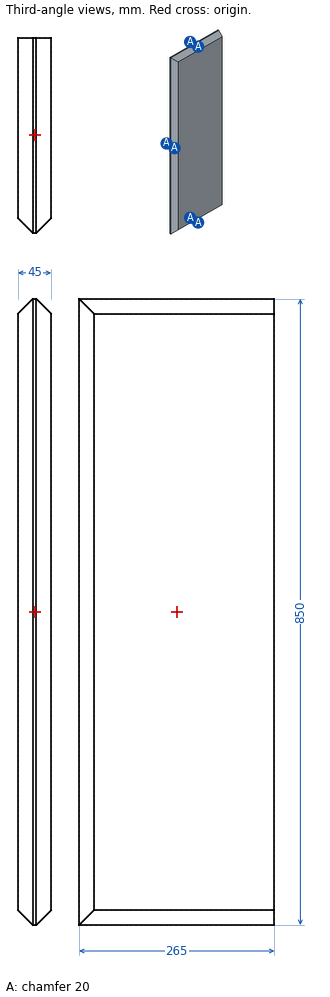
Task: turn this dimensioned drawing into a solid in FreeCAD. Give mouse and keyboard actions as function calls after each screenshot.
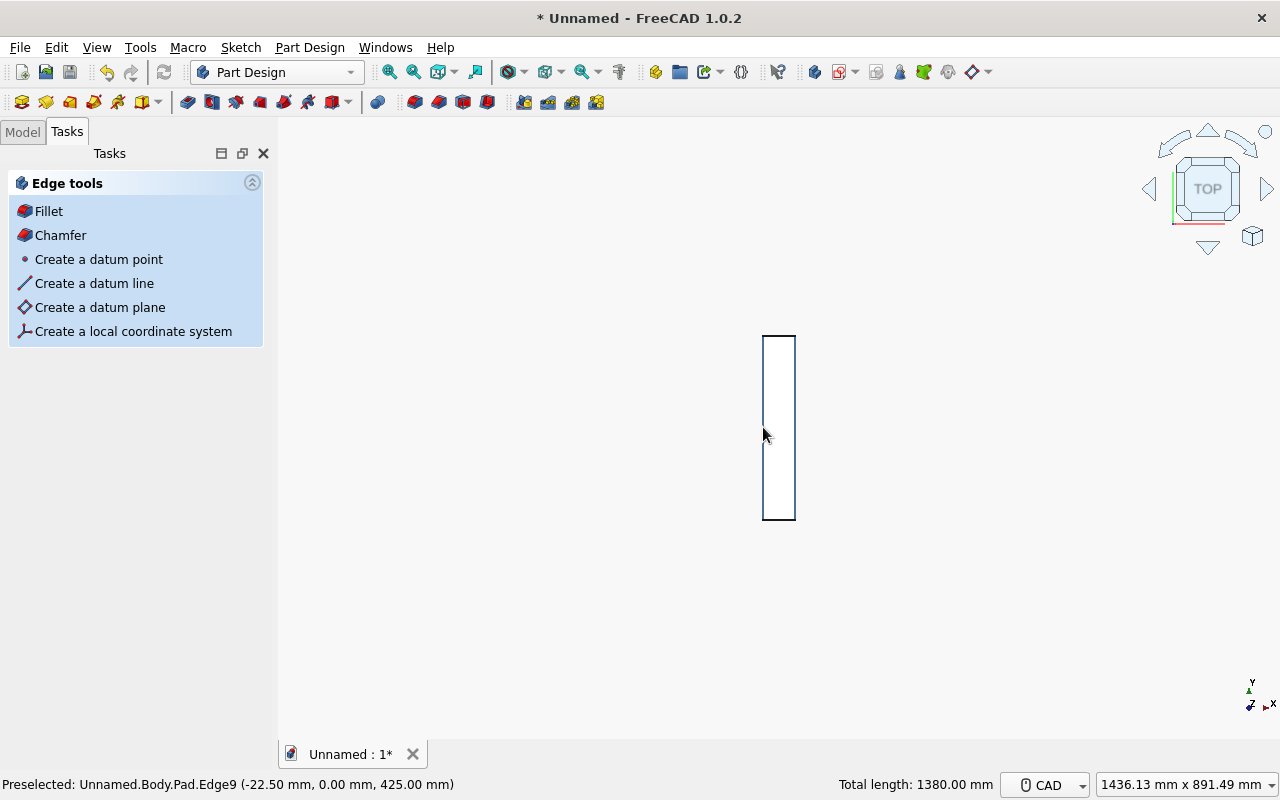
key(1)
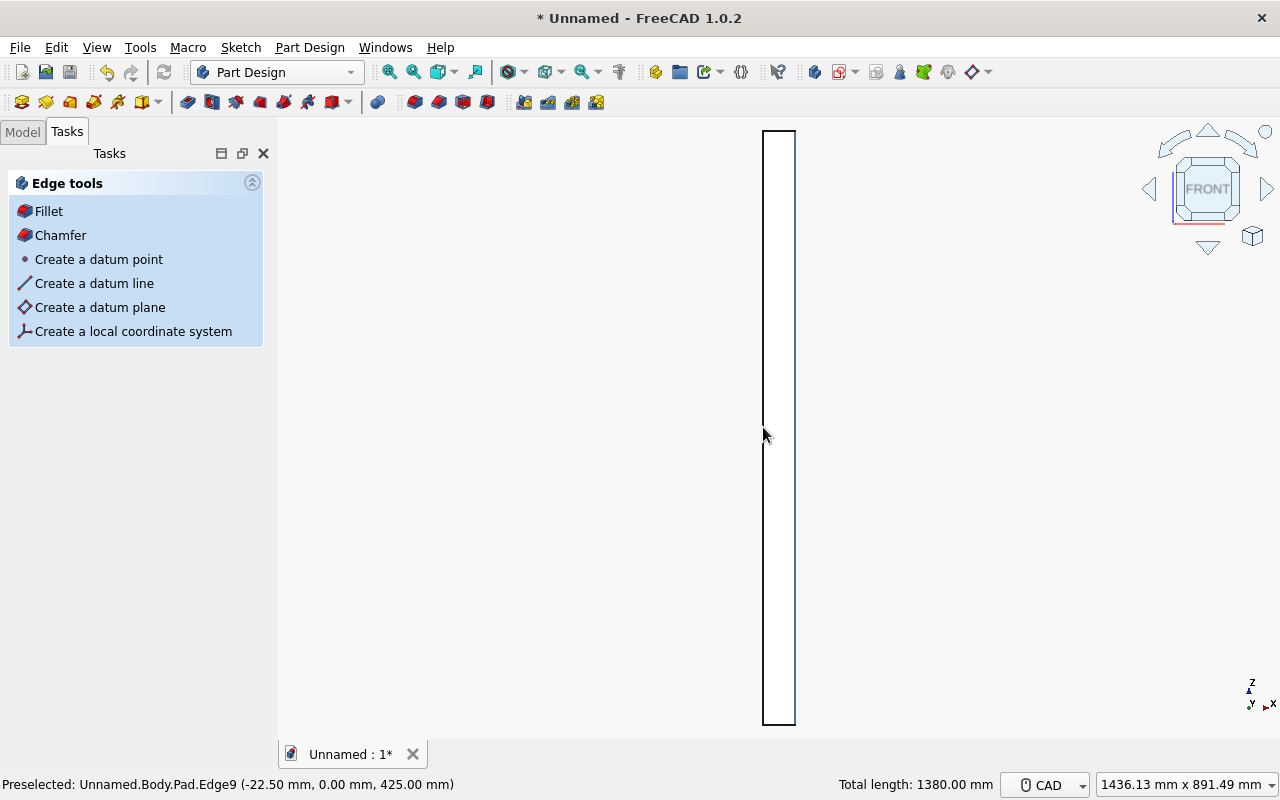
click(763, 427, ctrl)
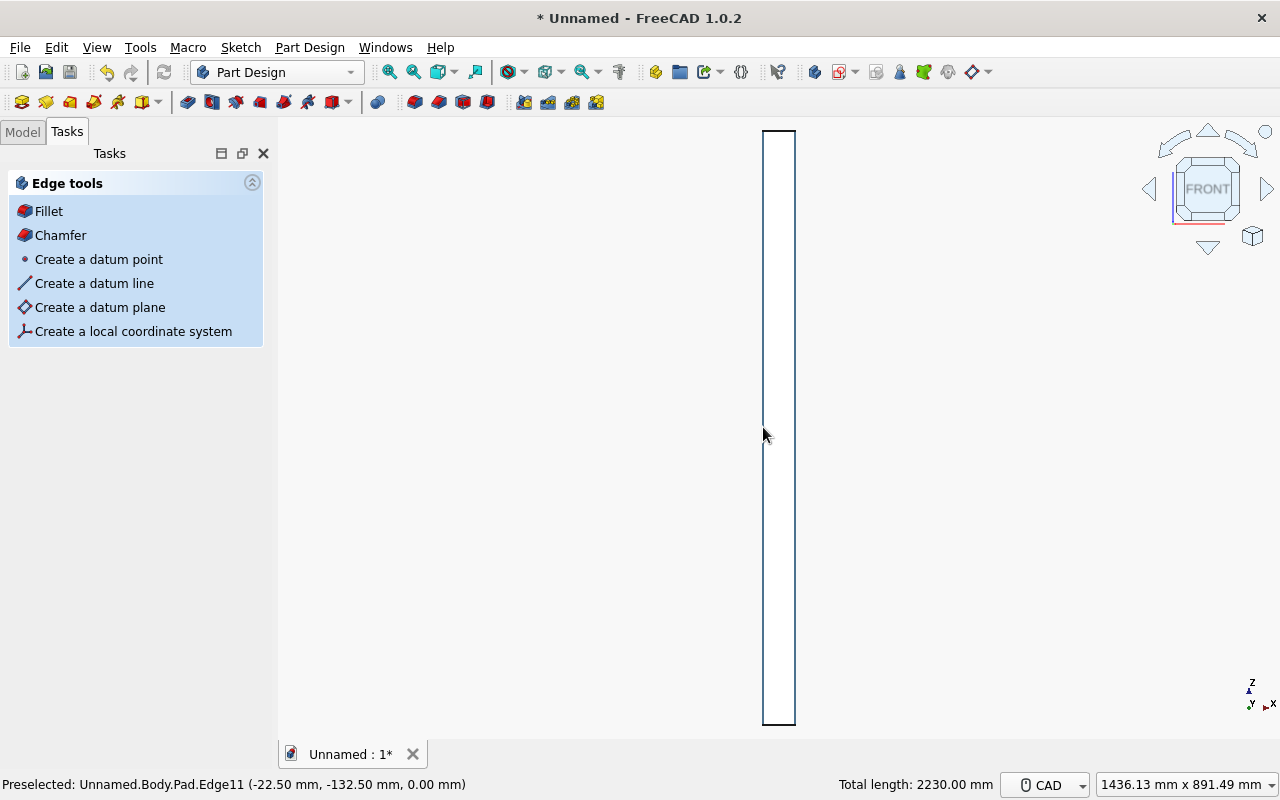
key(3)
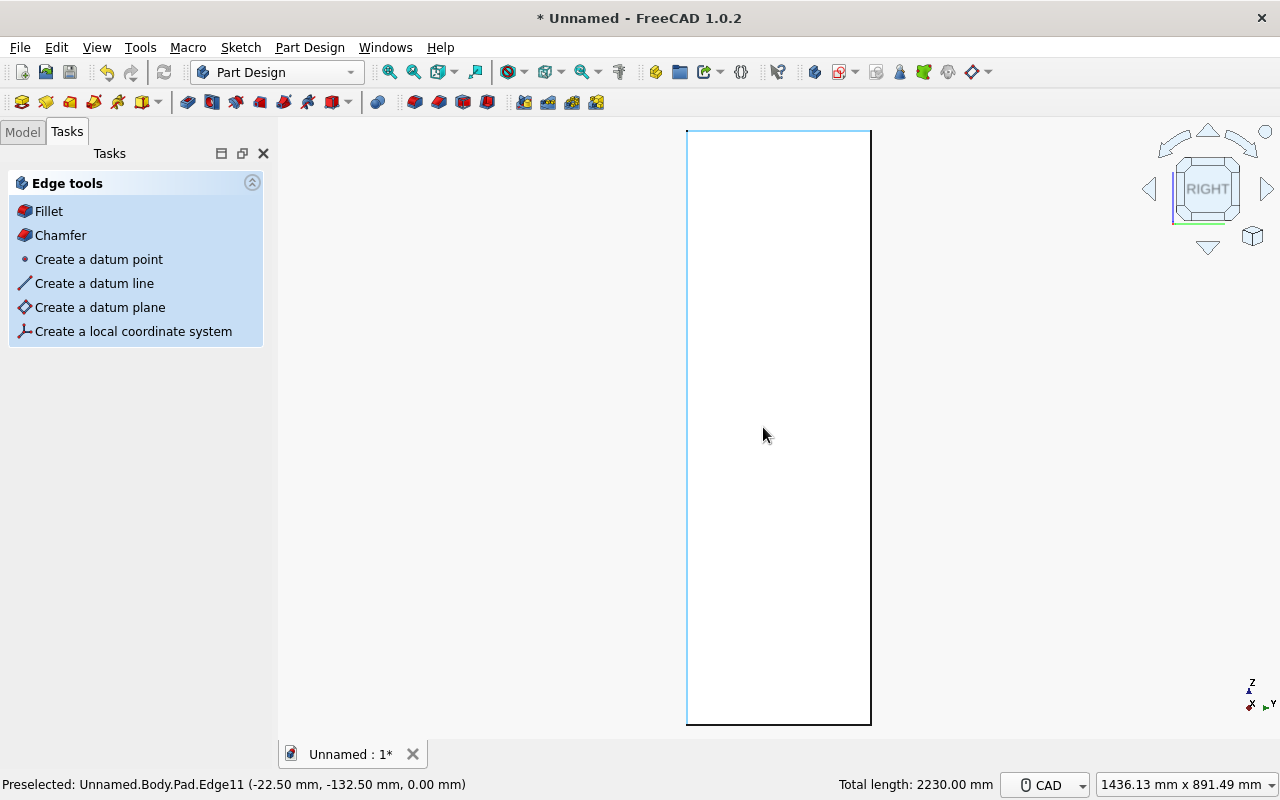
key(5)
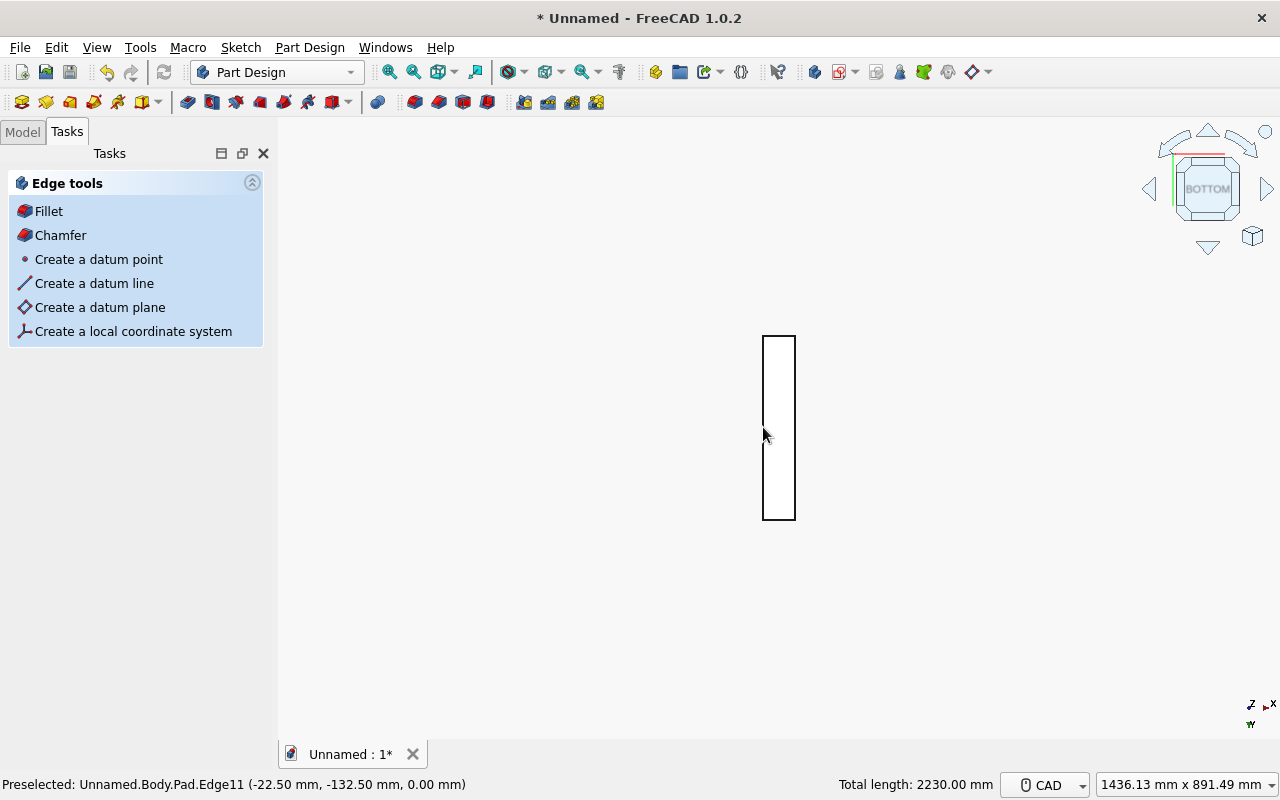
key(v)
key(f)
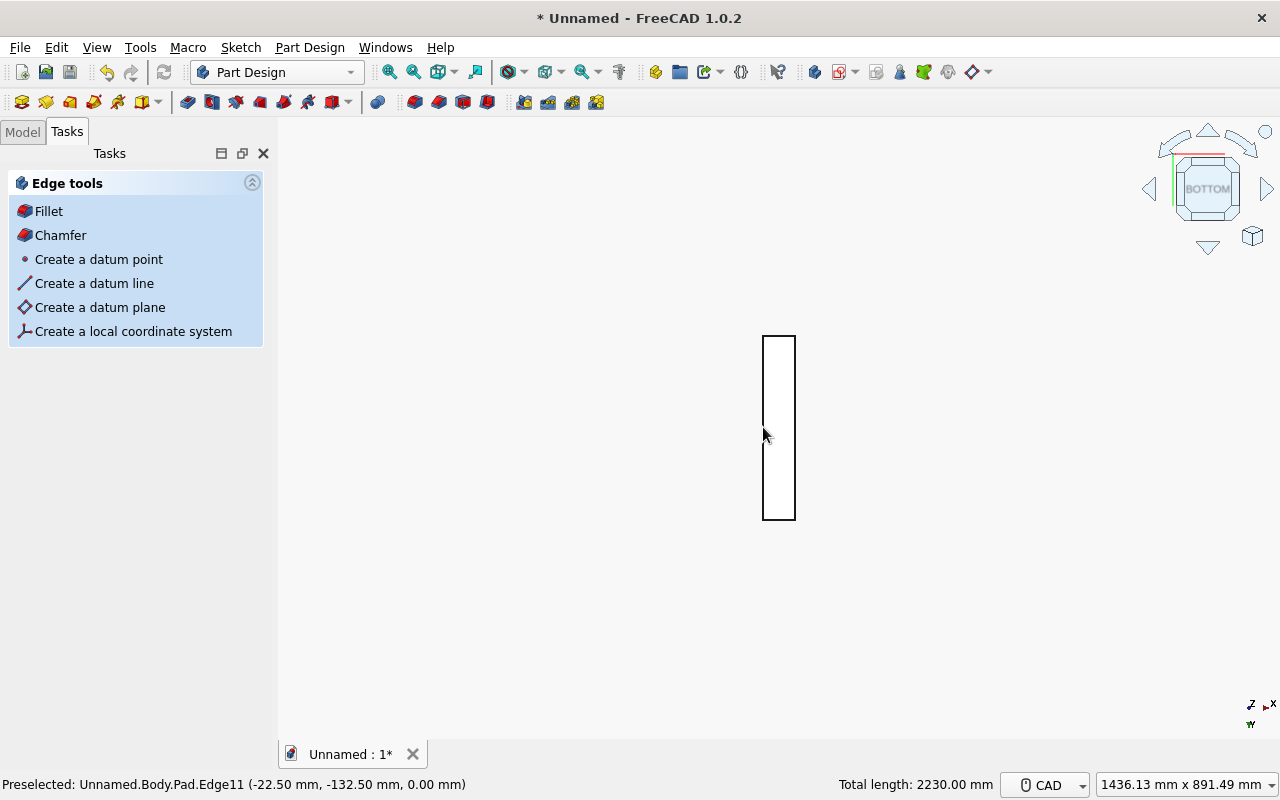
click(795, 427, ctrl)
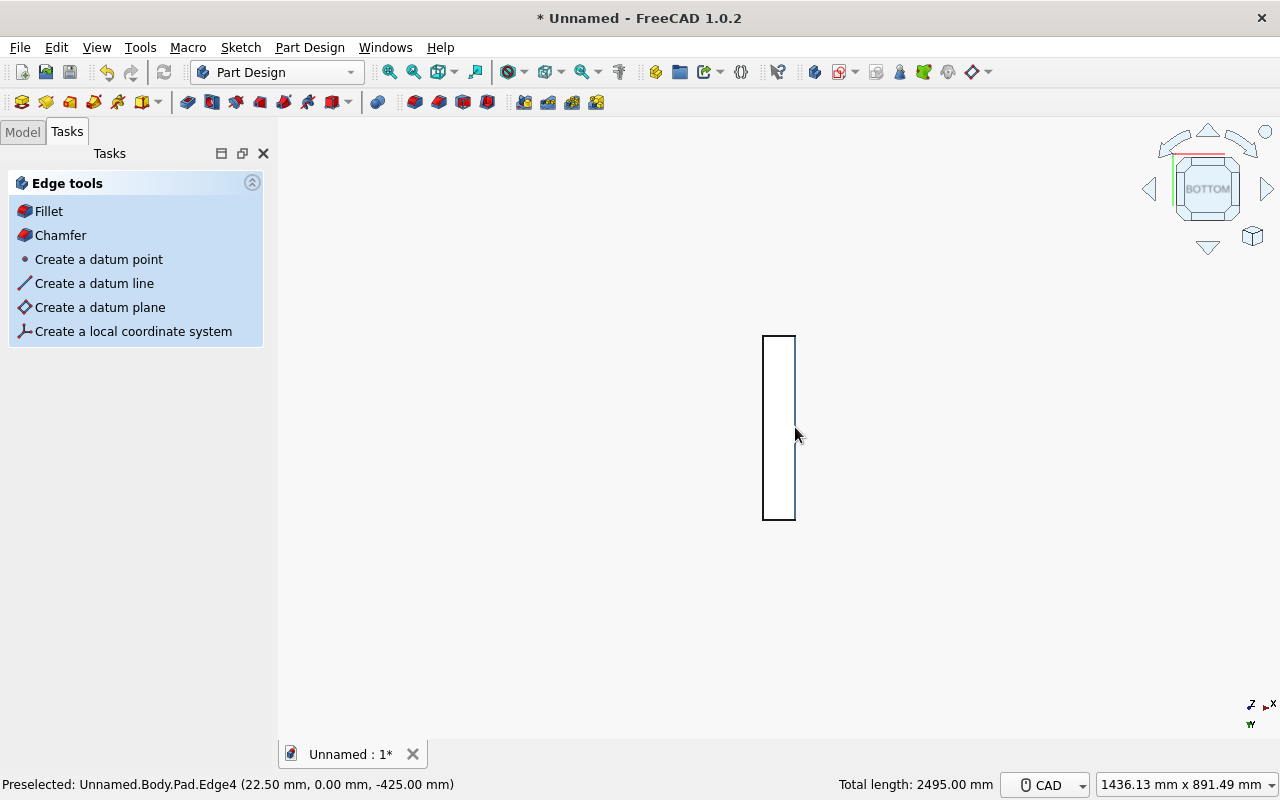
click(763, 427, ctrl)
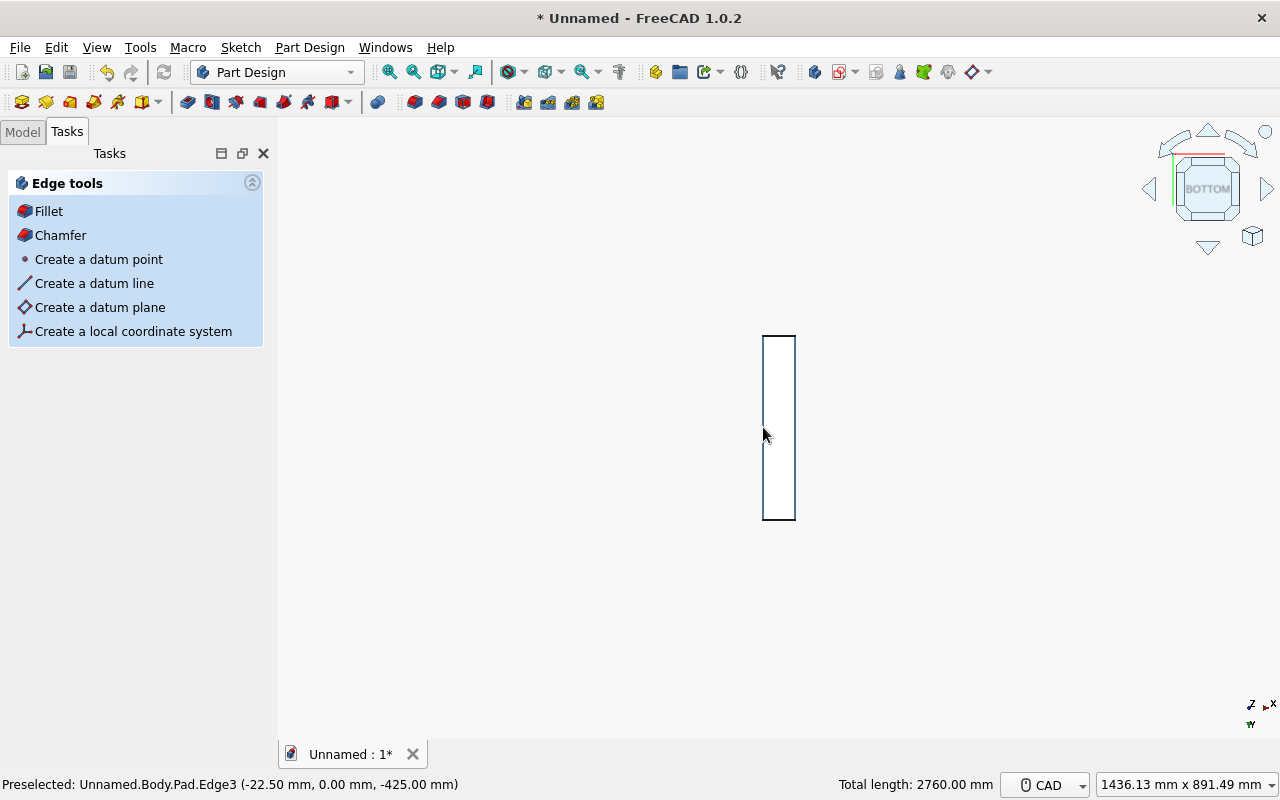
click(440, 102)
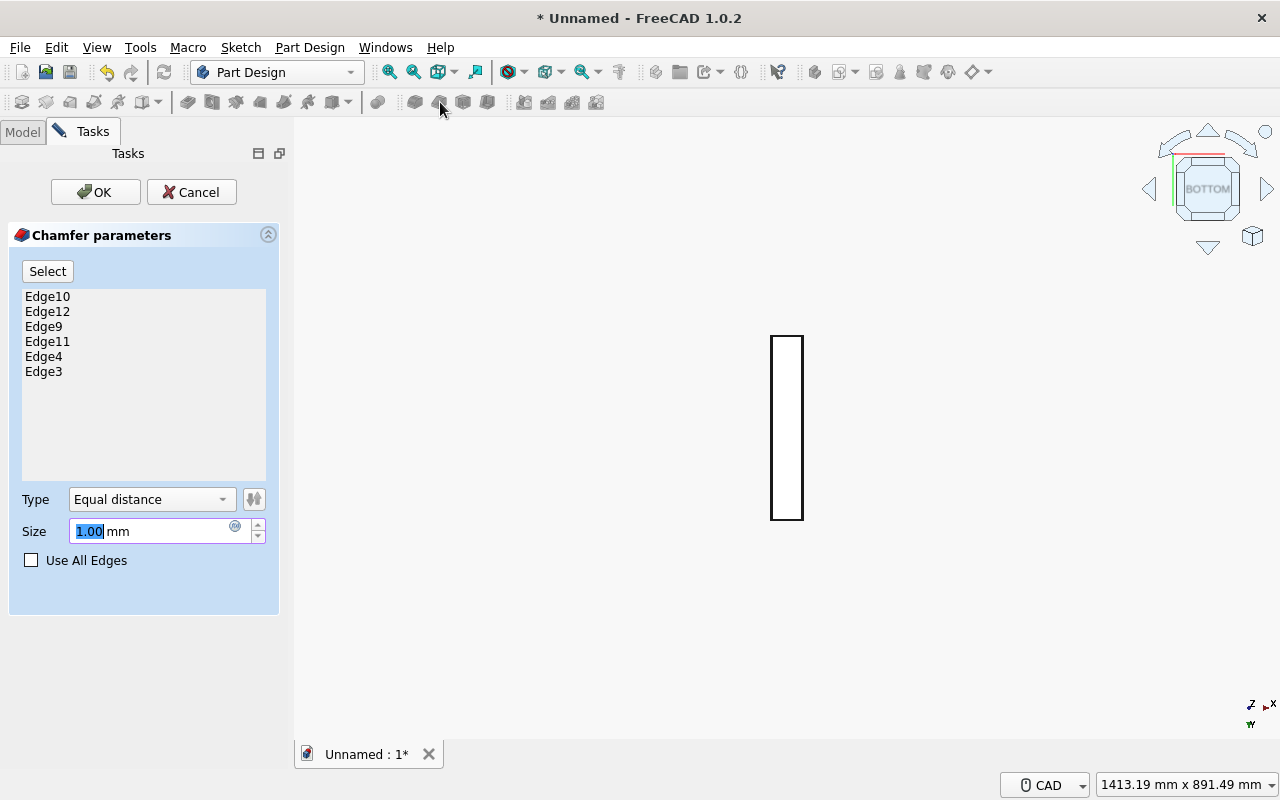
text(20)
key(Tab)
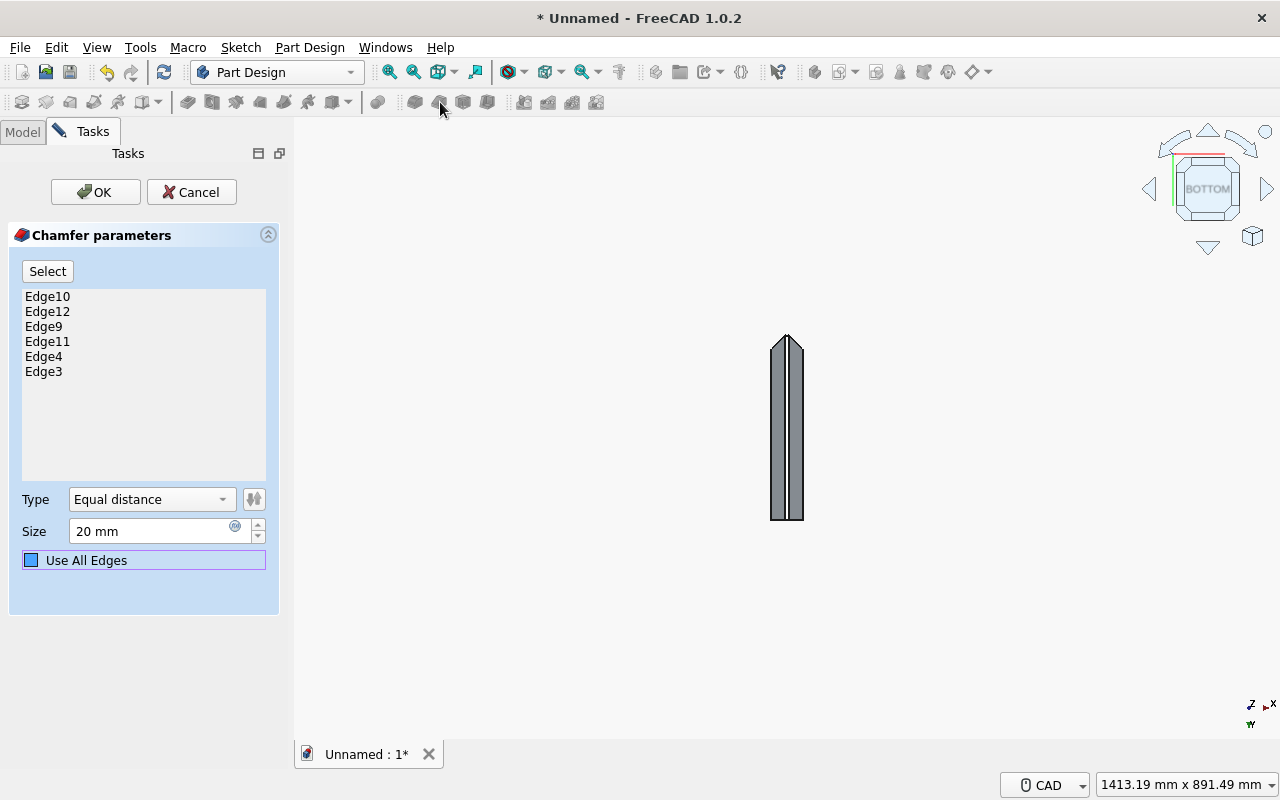
click(96, 192)